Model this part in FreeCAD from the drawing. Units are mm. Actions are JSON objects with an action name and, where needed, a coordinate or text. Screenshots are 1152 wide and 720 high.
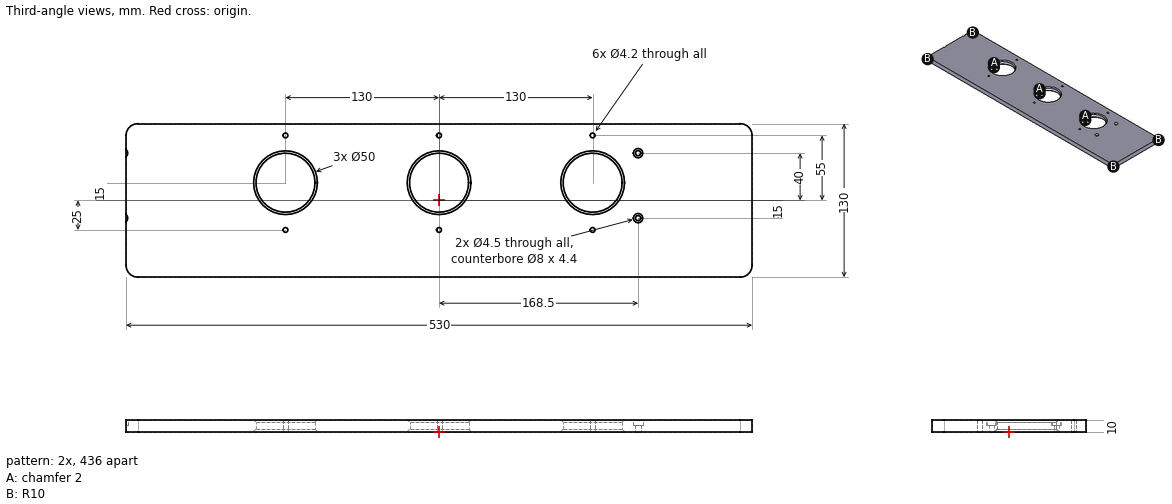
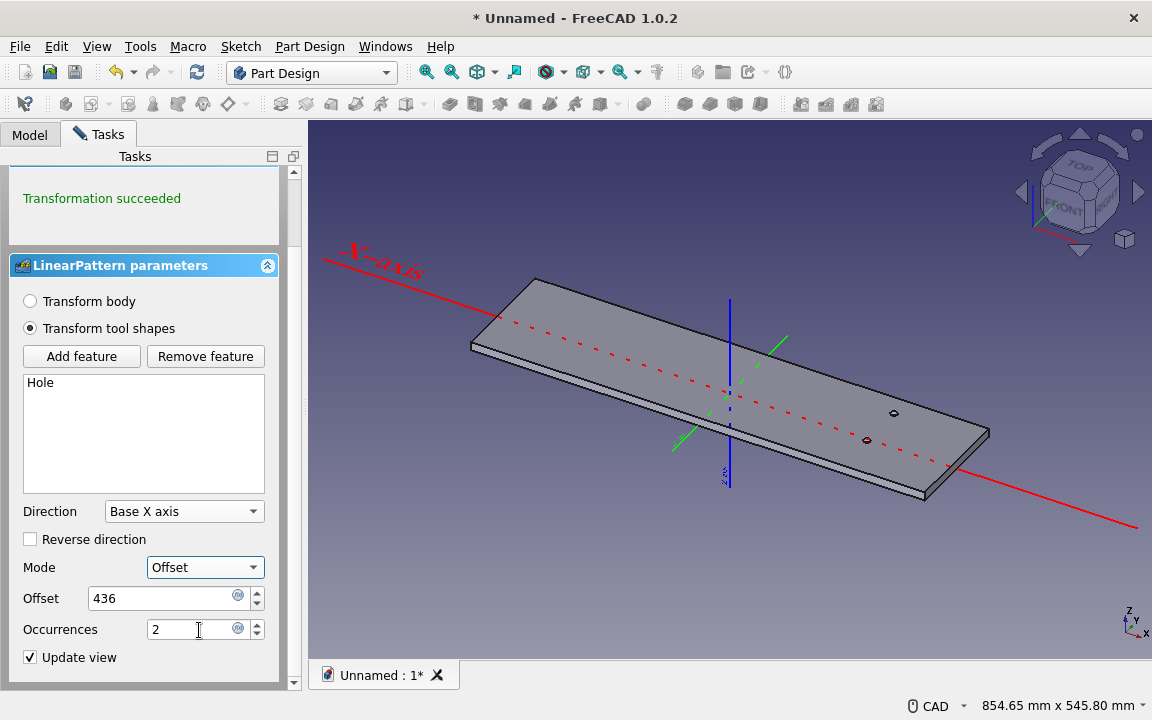
{"action": "left_click", "coordinate": [31, 539]}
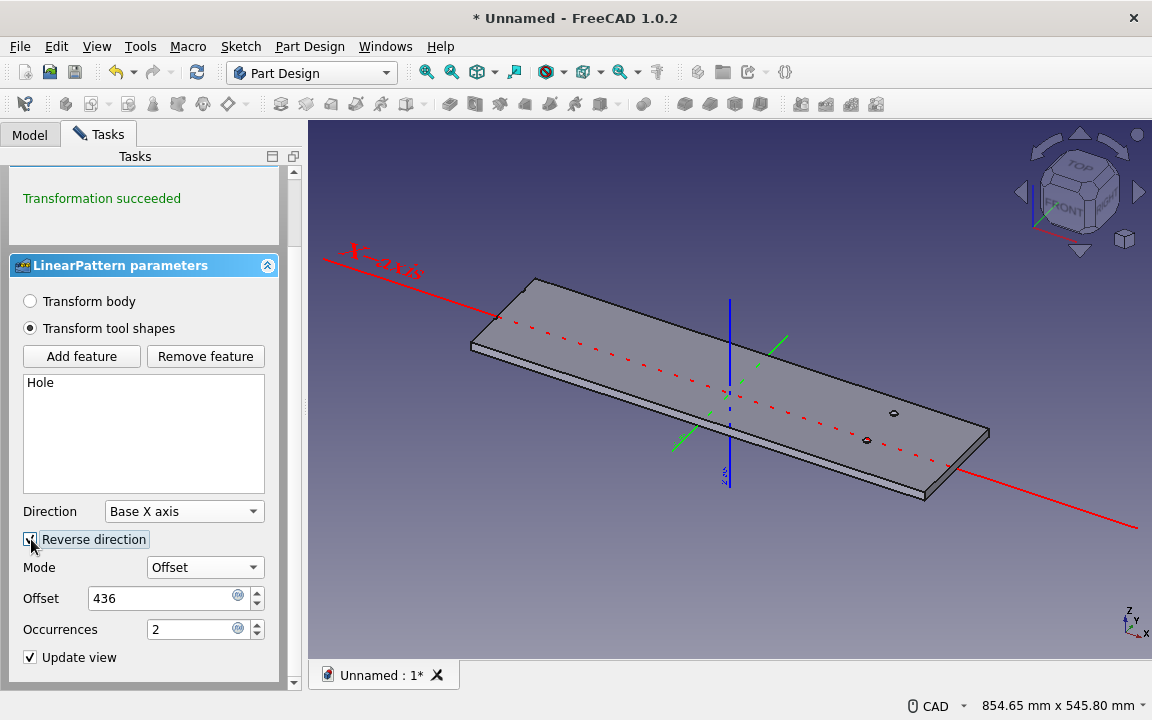
{"action": "scroll", "coordinate": [294, 428], "scroll_direction": "up", "scroll_amount": 3}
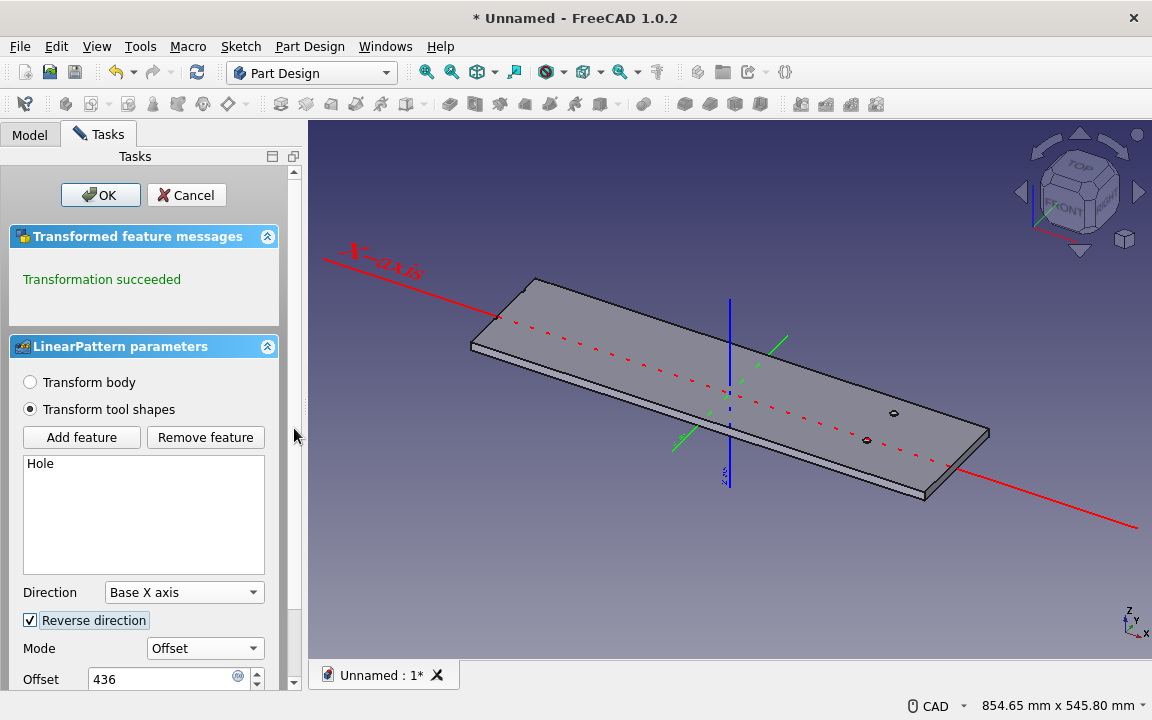
{"action": "left_click", "coordinate": [101, 195]}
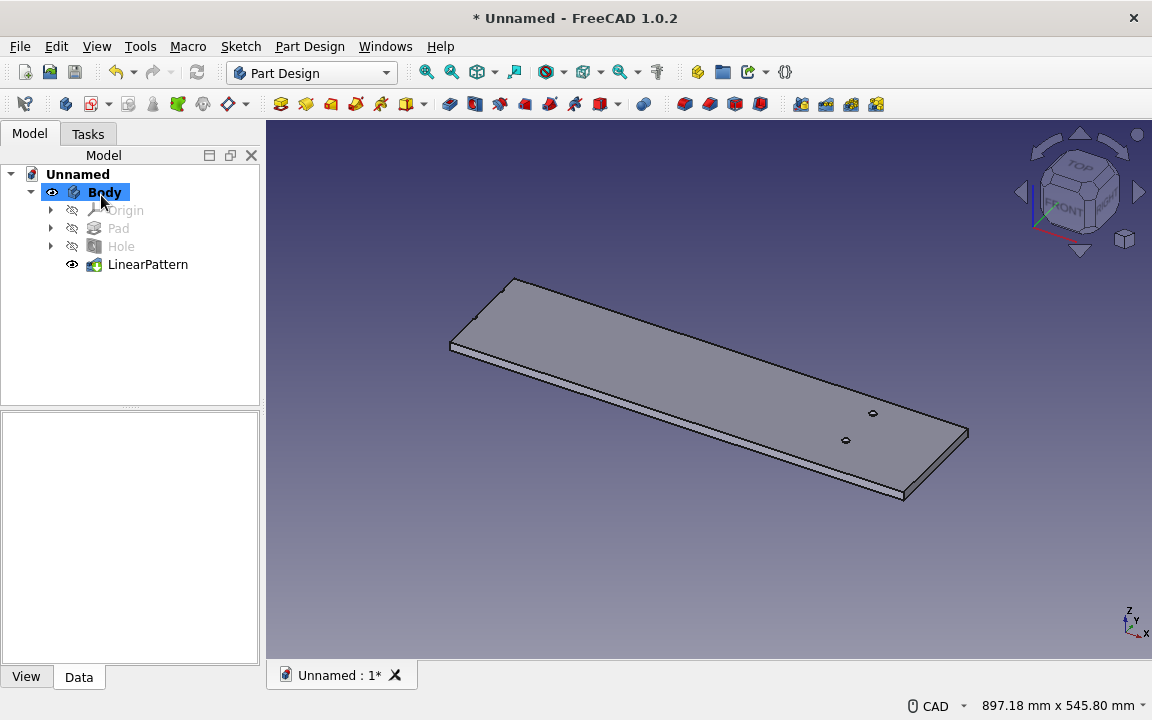
{"action": "left_click", "coordinate": [774, 406]}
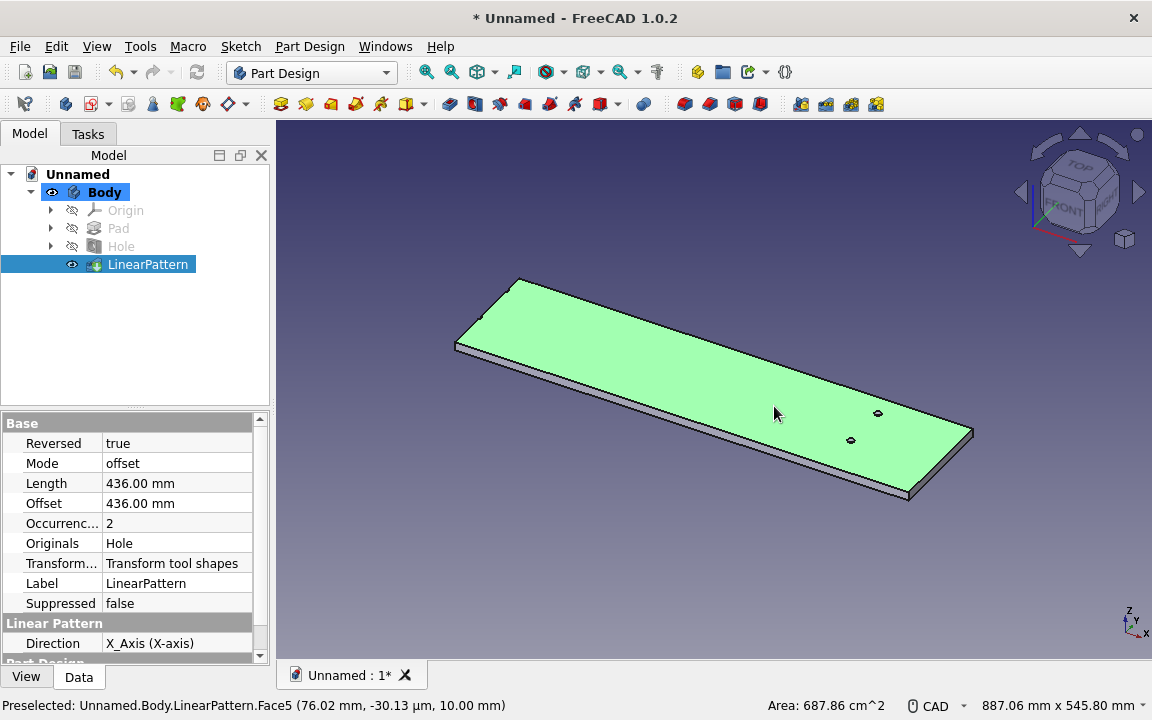
{"action": "left_click", "coordinate": [90, 104]}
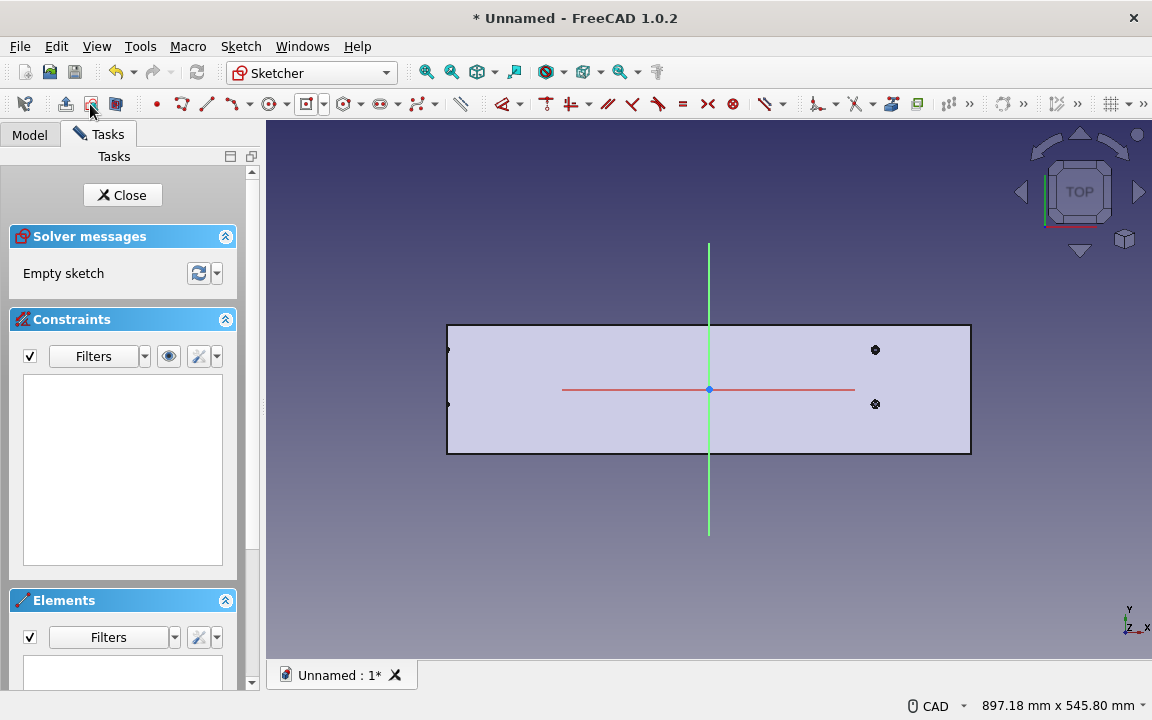
{"action": "scroll", "coordinate": [848, 345], "scroll_direction": "up", "scroll_amount": 2}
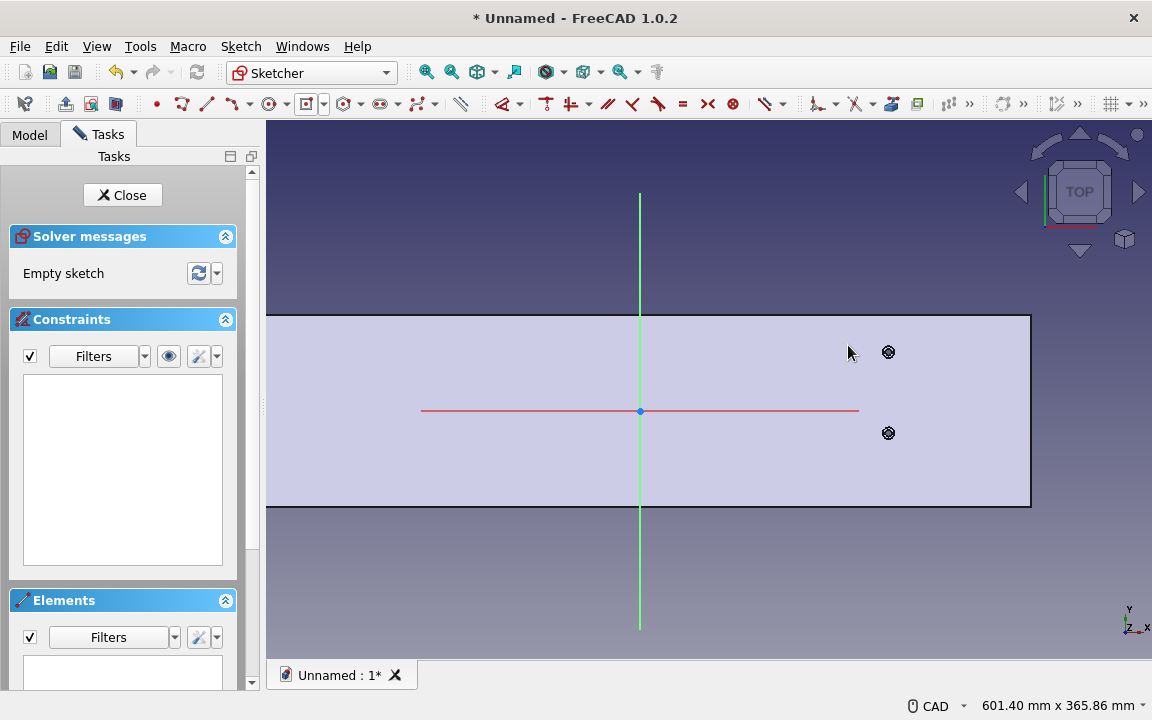
{"action": "left_click", "coordinate": [268, 104]}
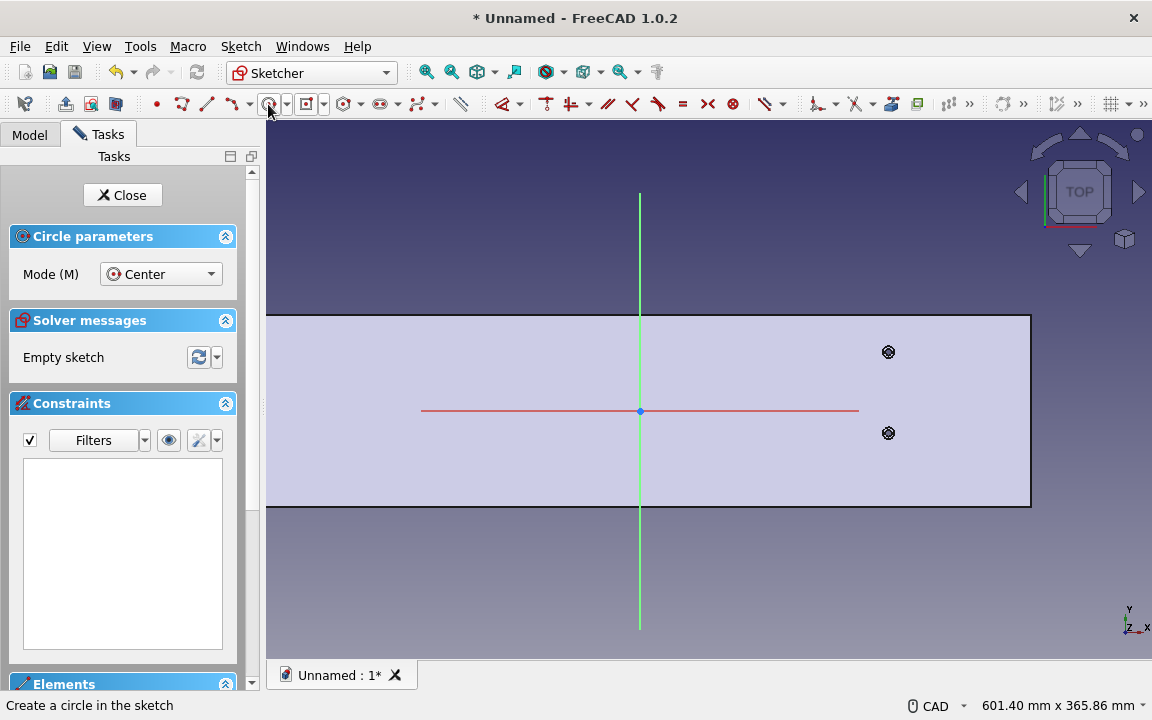
{"action": "left_click", "coordinate": [449, 389]}
{"action": "mouse_move", "coordinate": [475, 363]}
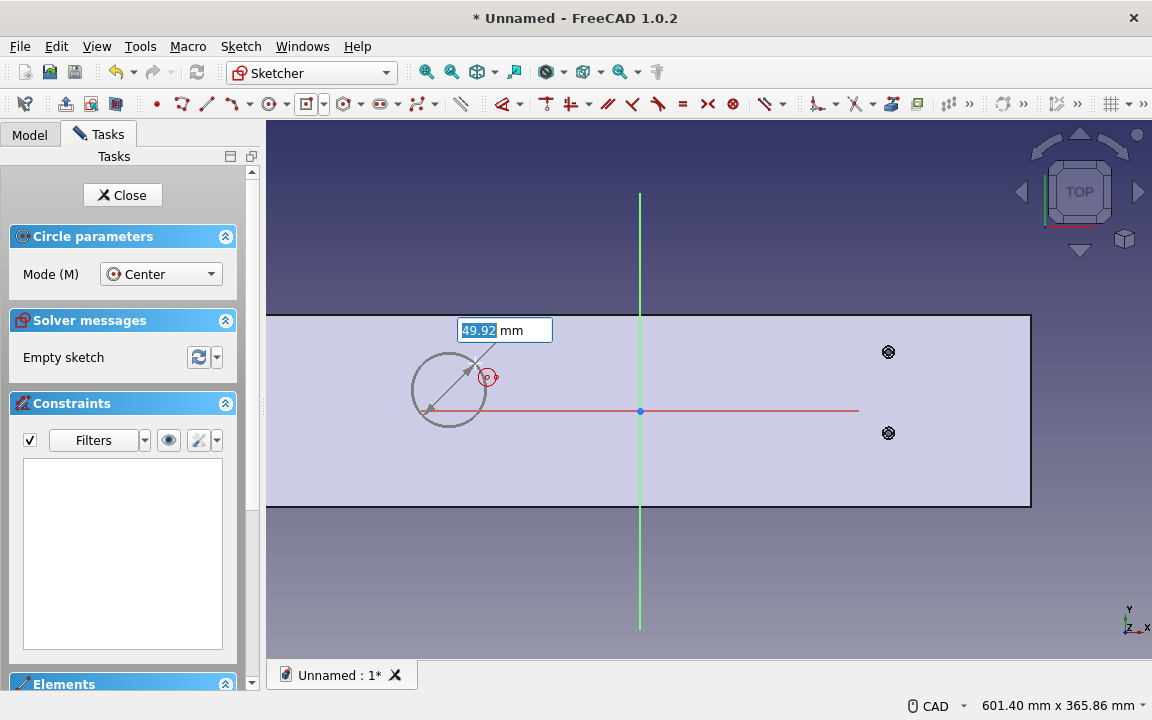
{"action": "type", "text": "50"}
{"action": "key", "text": "Return"}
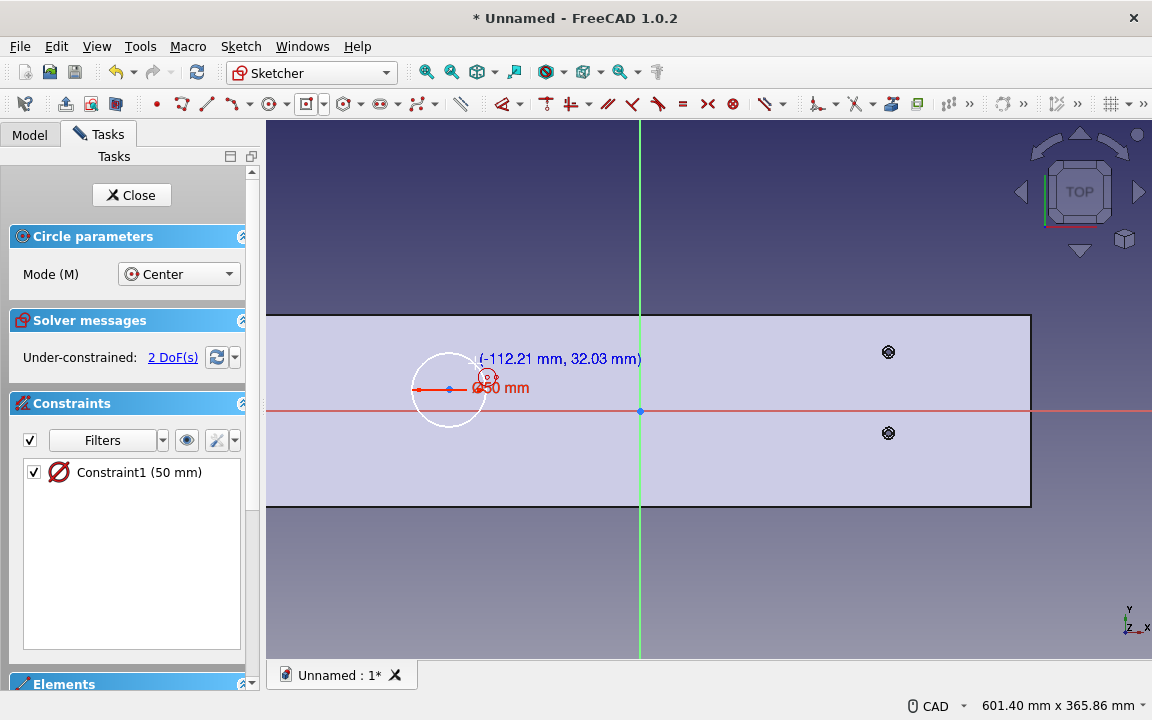
{"action": "left_click", "coordinate": [640, 389]}
{"action": "mouse_move", "coordinate": [666, 363]}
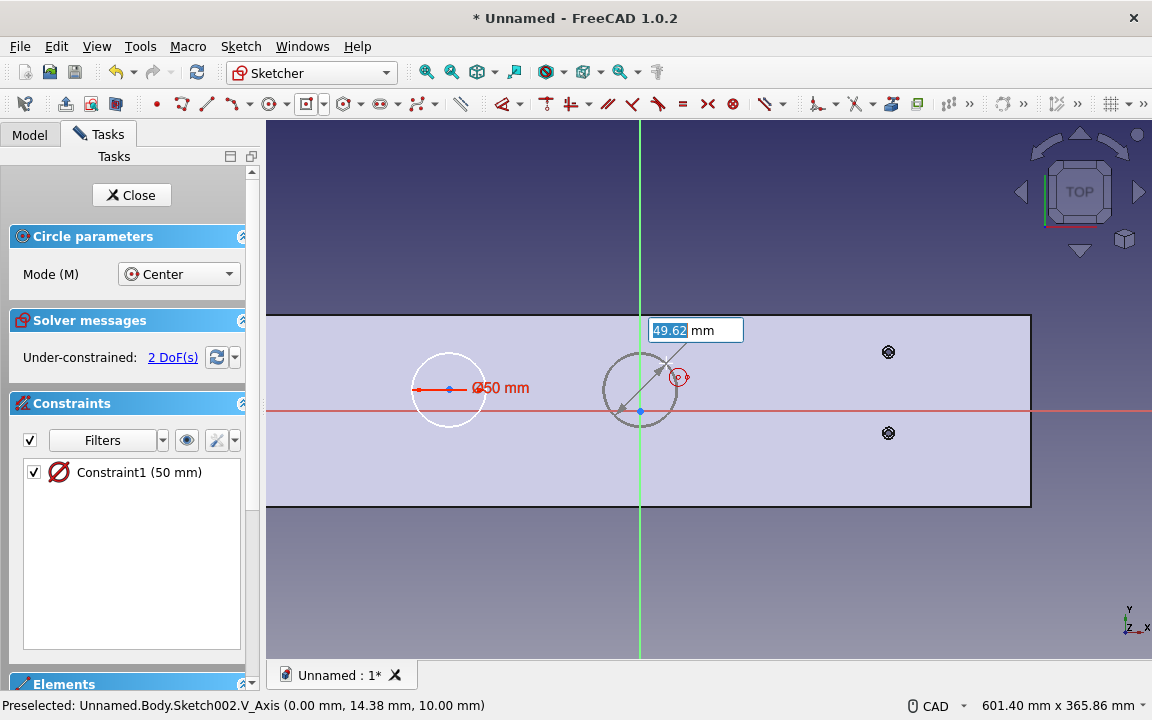
{"action": "type", "text": "50"}
{"action": "key", "text": "Return"}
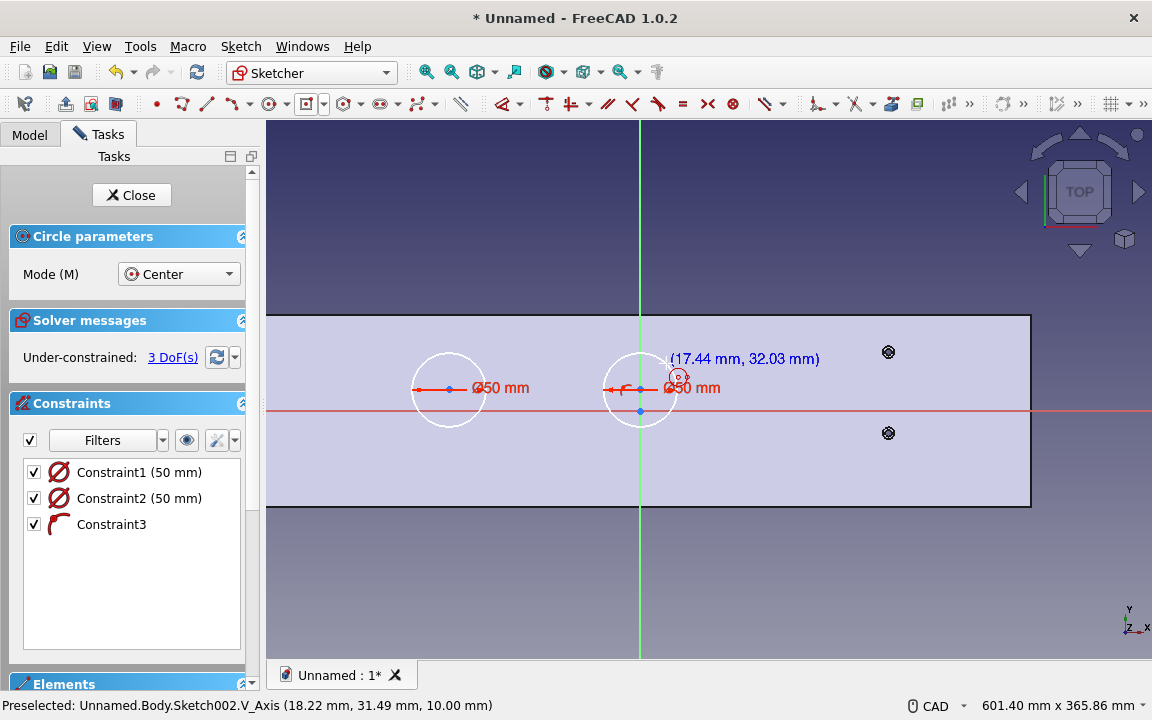
{"action": "left_click", "coordinate": [832, 389]}
{"action": "mouse_move", "coordinate": [858, 363]}